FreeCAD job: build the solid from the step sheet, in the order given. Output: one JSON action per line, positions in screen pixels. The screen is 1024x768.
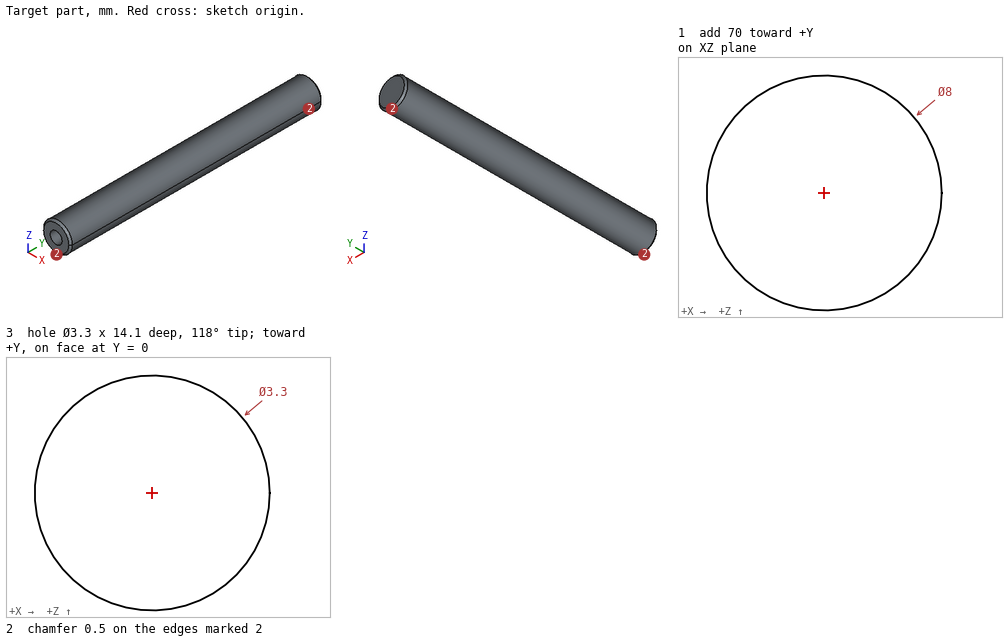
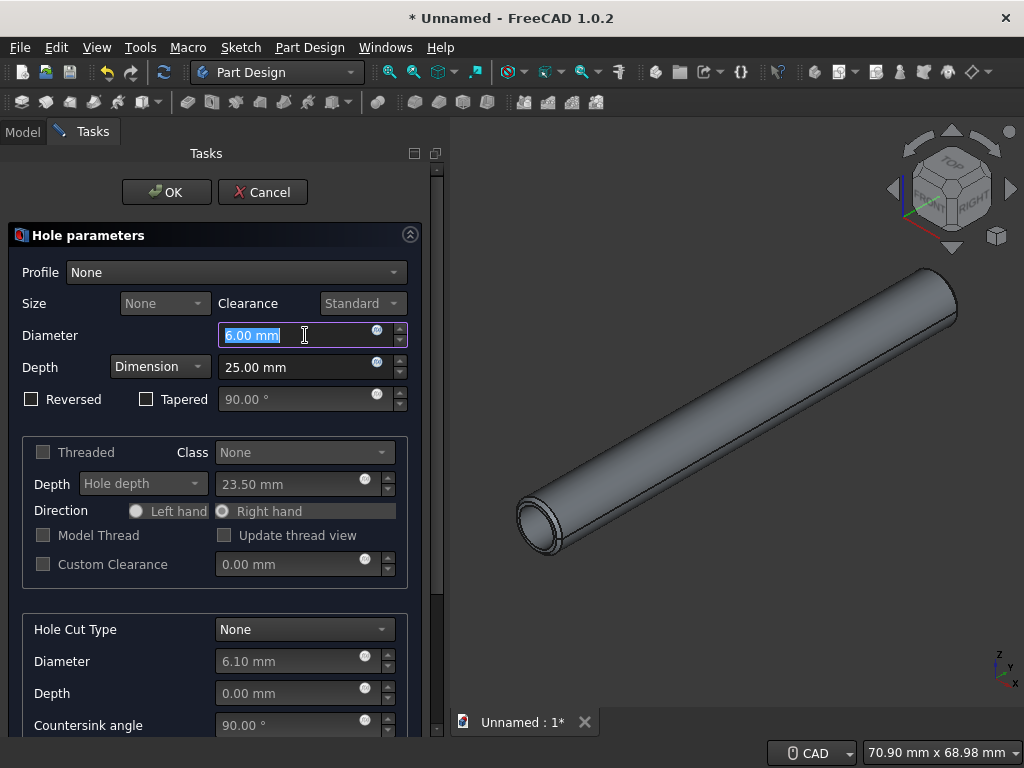
{"action": "type", "text": "3.3"}
{"action": "key", "text": "Tab"}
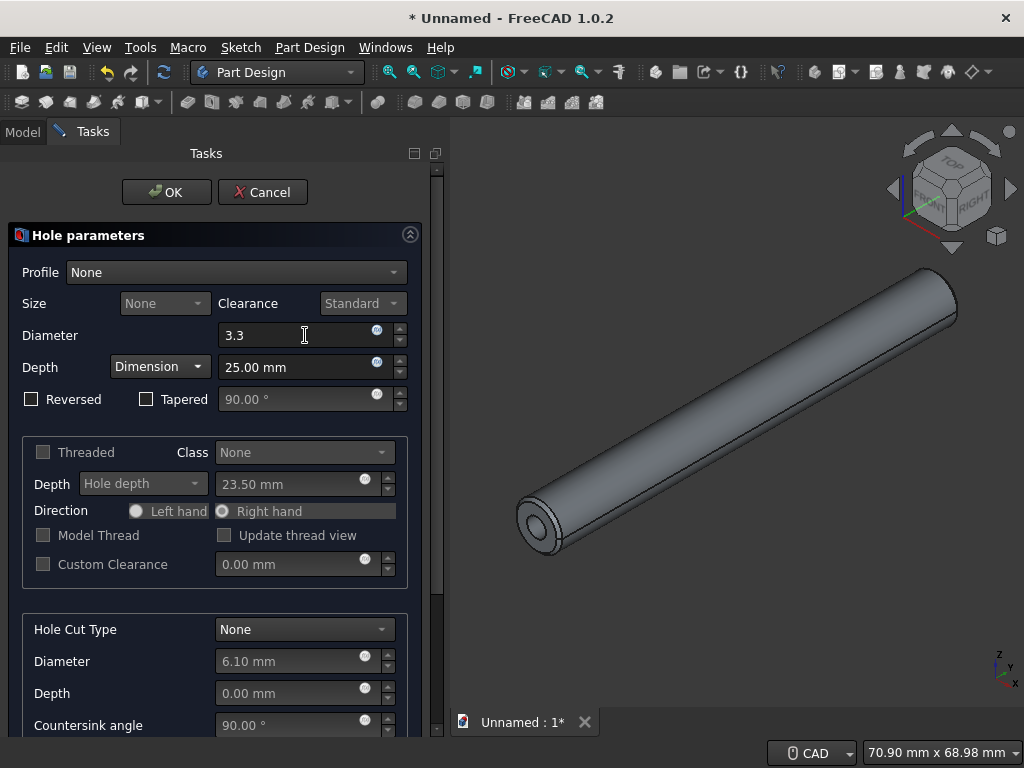
{"action": "triple_click", "coordinate": [305, 367]}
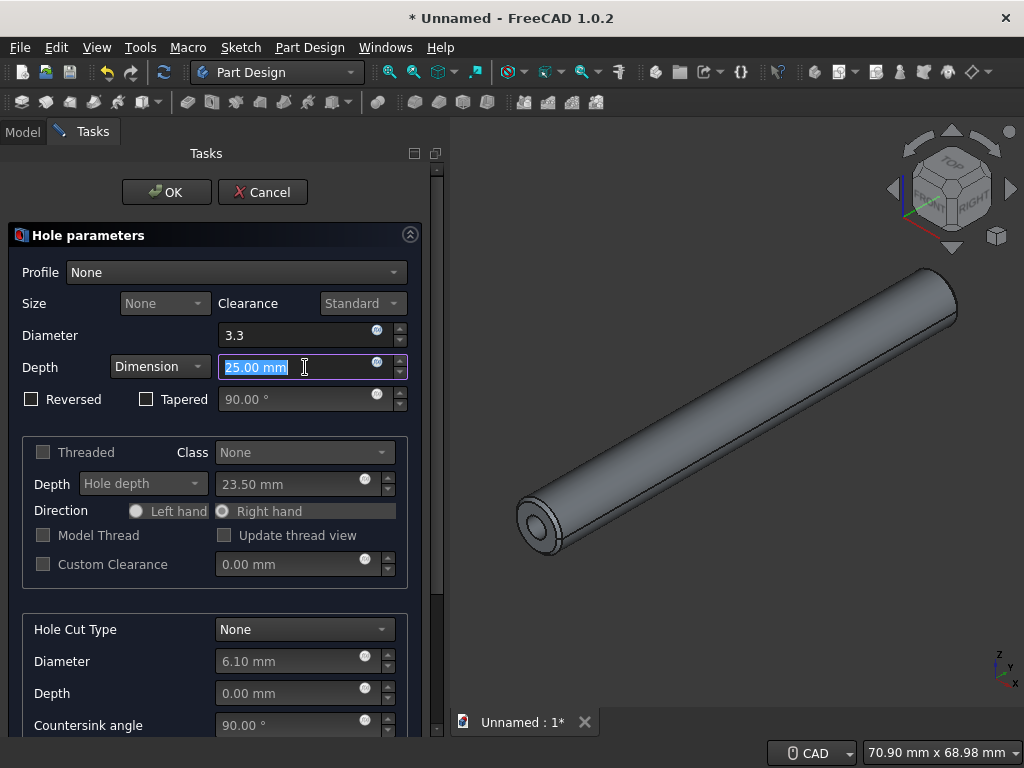
{"action": "type", "text": "14.1"}
{"action": "key", "text": "Tab"}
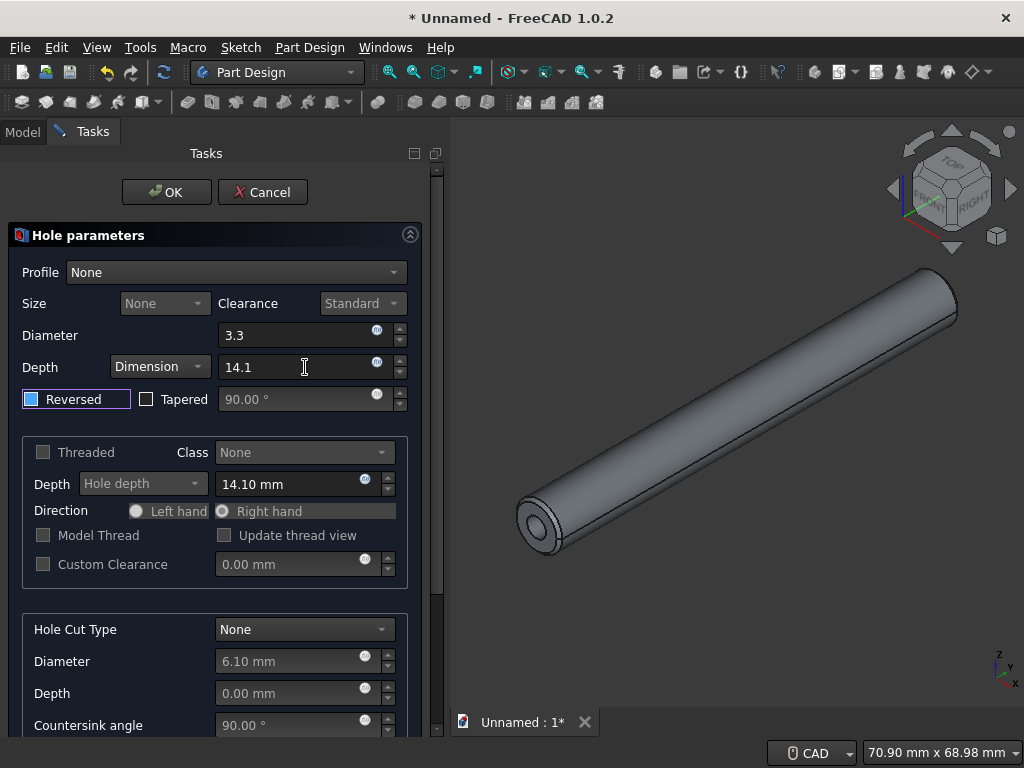
{"action": "left_click", "coordinate": [167, 192]}